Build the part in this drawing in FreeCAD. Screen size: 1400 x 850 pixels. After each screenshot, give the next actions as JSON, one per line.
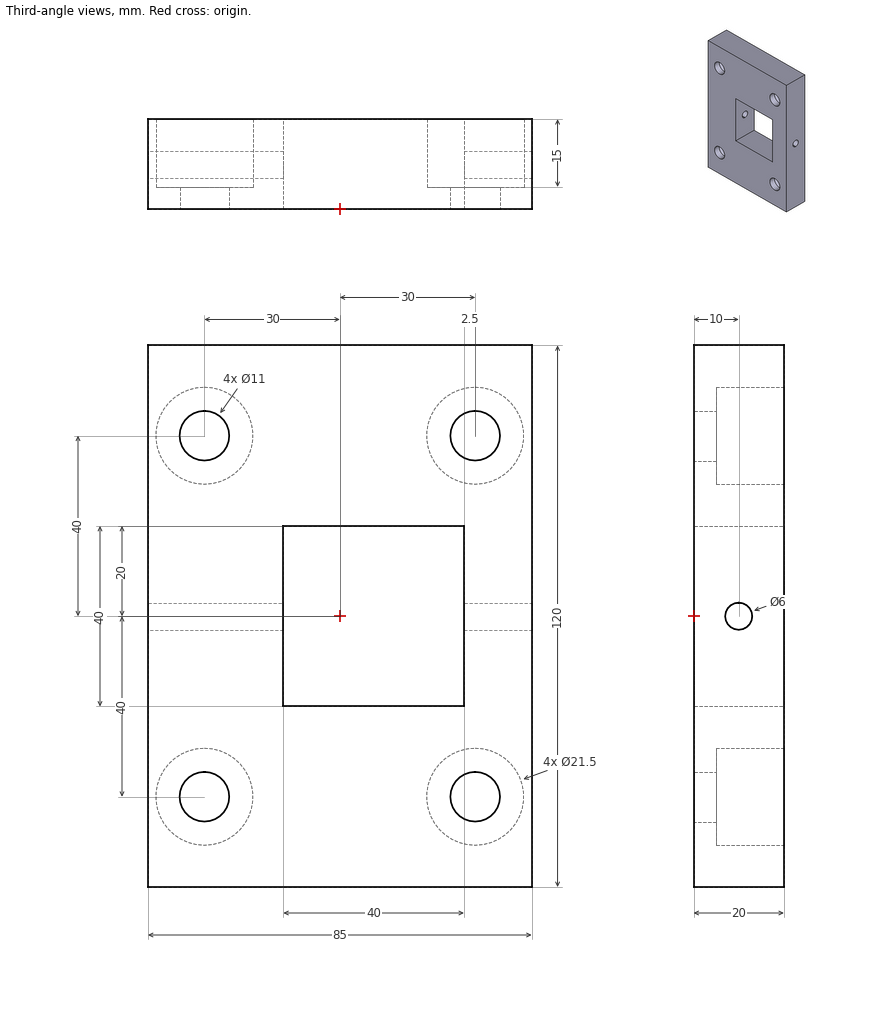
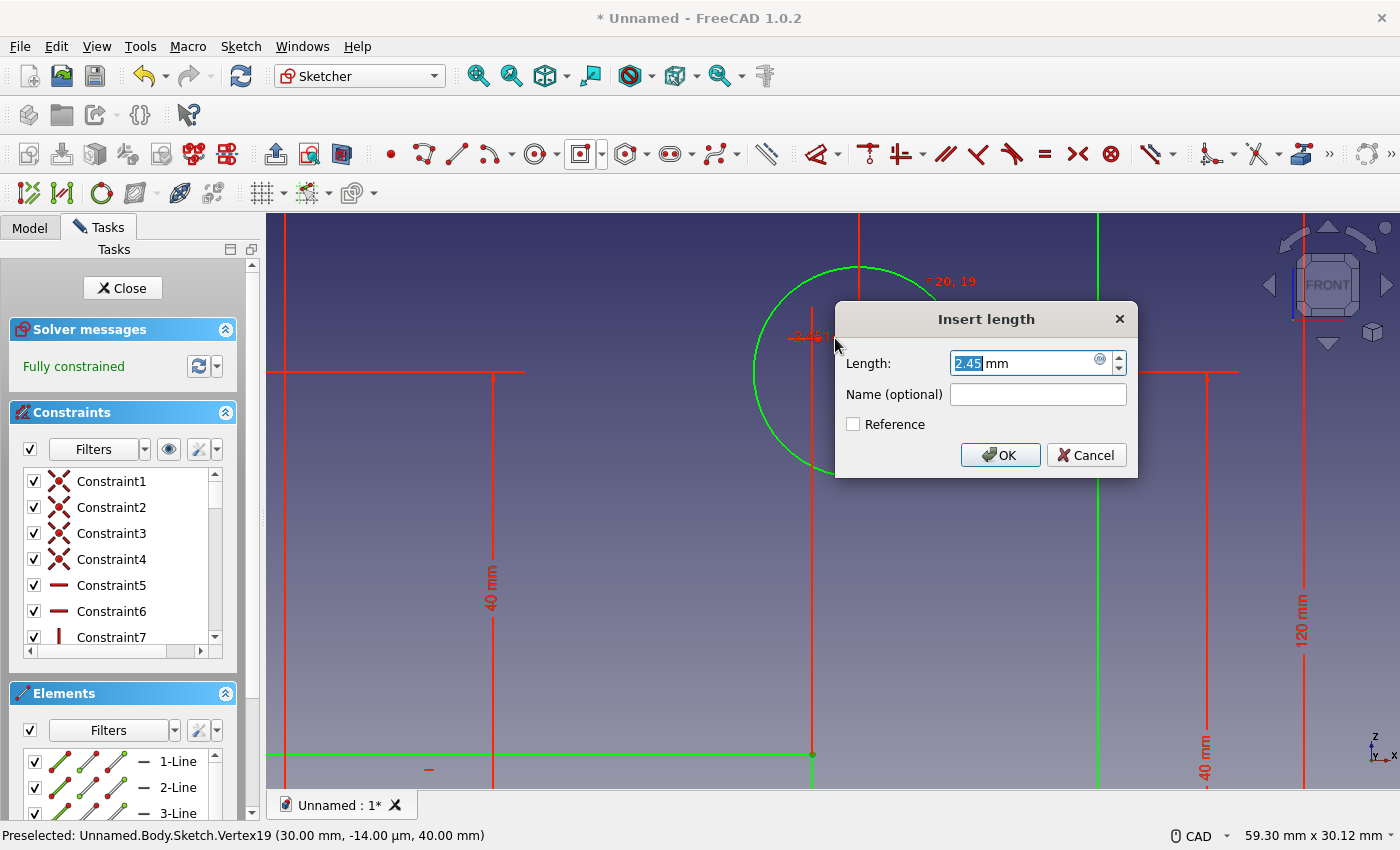
{"action": "type", "text": "2.5"}
{"action": "key", "text": "Return"}
{"action": "key", "text": "Escape"}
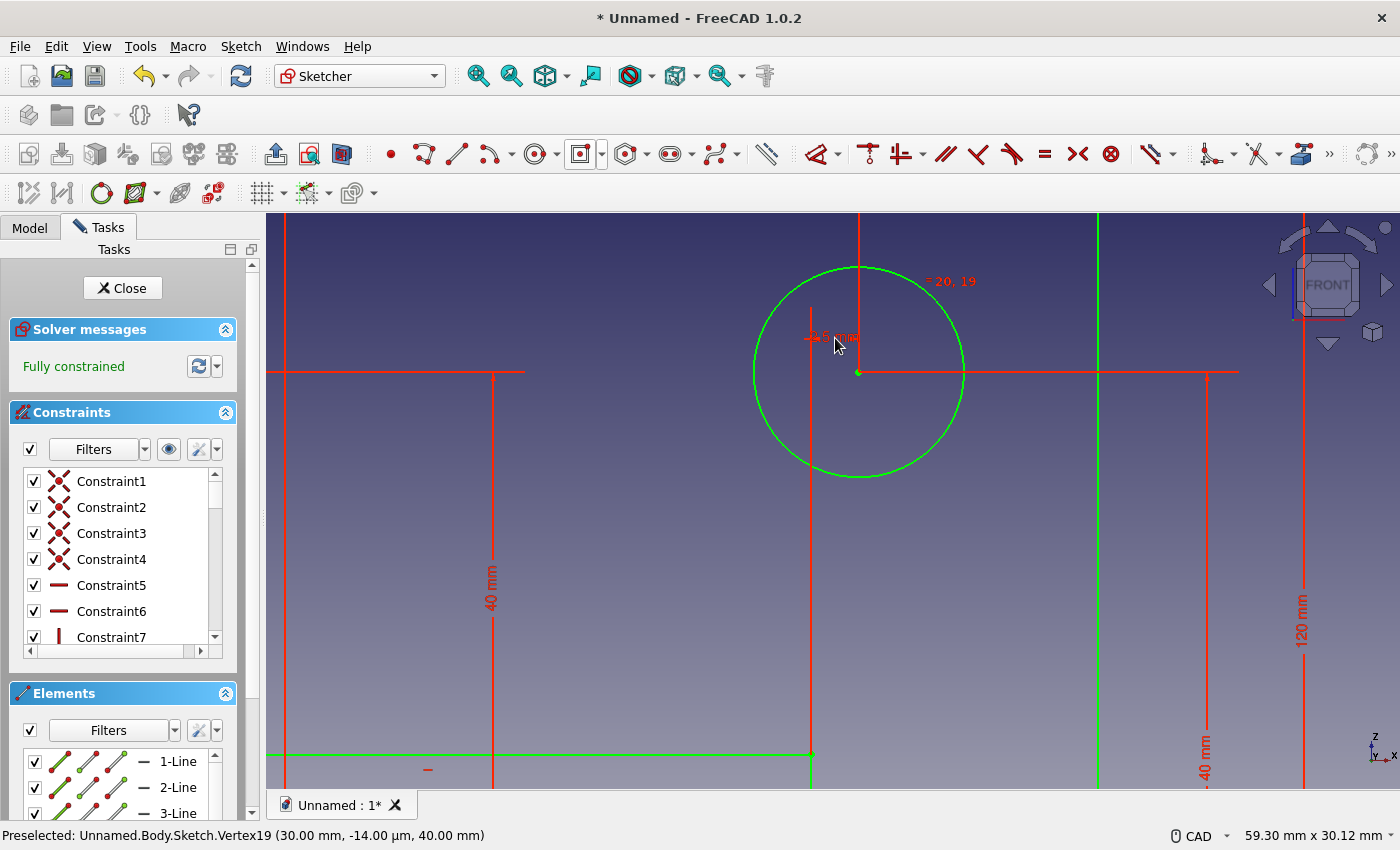
{"action": "left_click", "coordinate": [123, 288]}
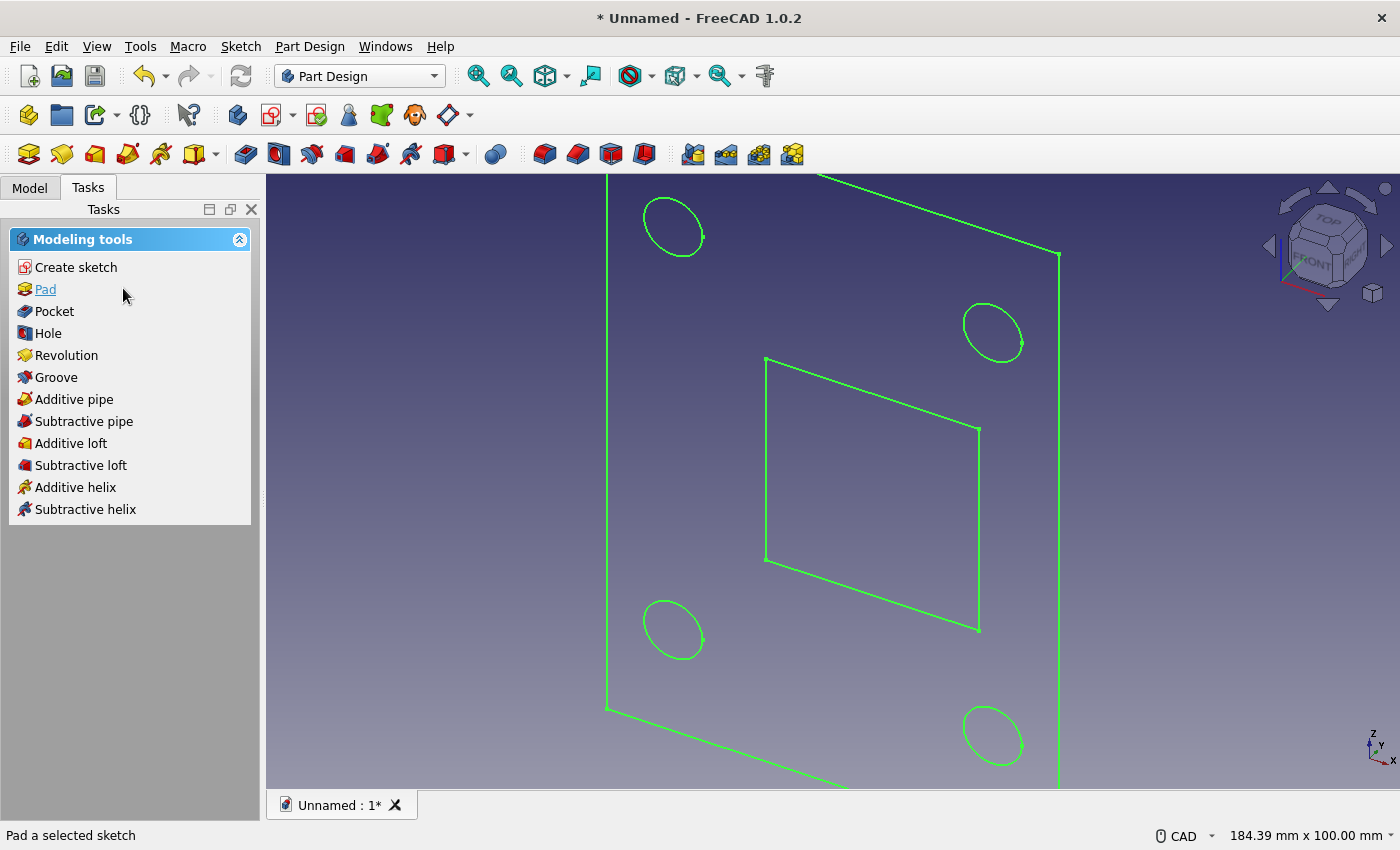
{"action": "left_click", "coordinate": [29, 154]}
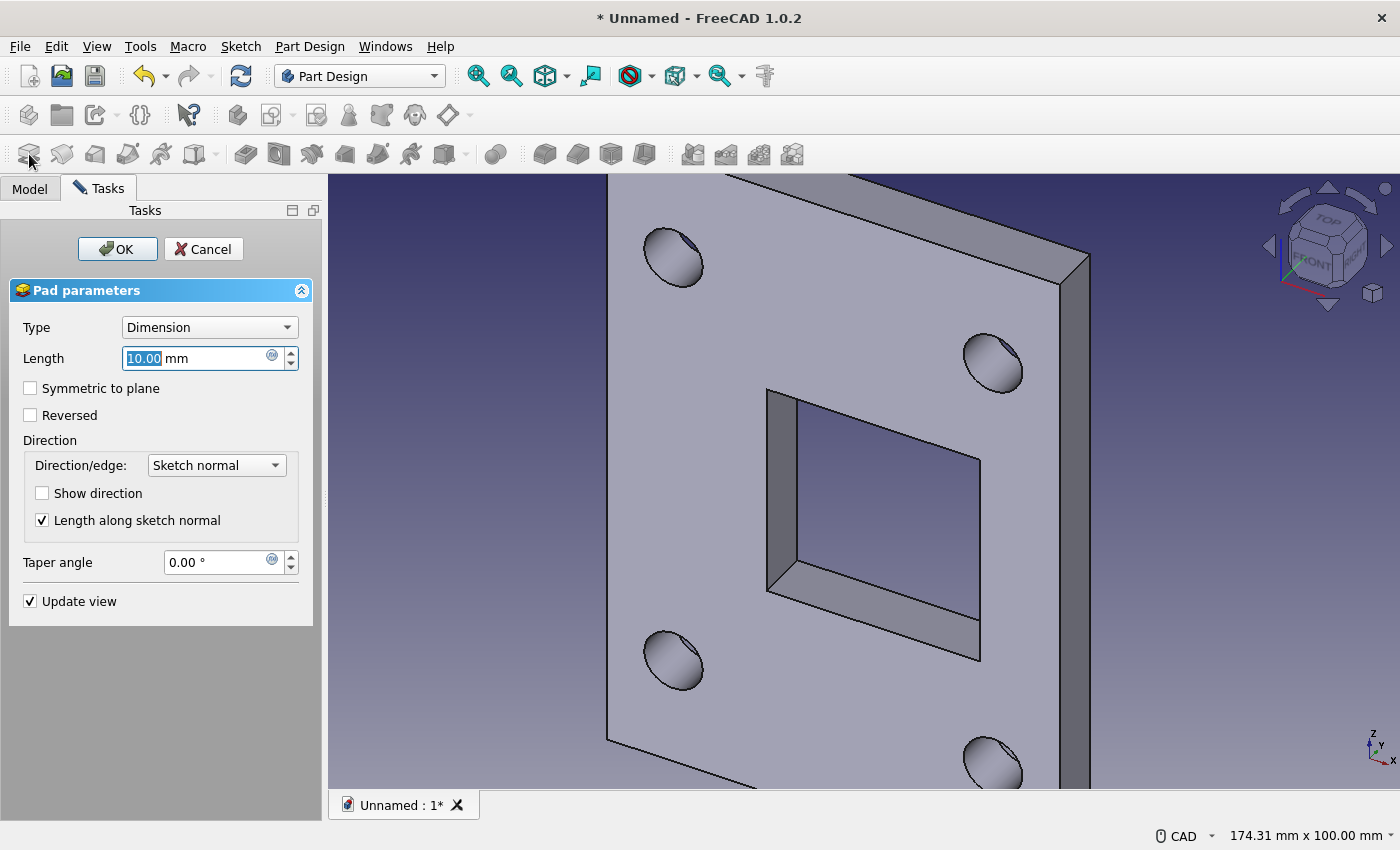
{"action": "type", "text": "20"}
{"action": "key", "text": "Tab"}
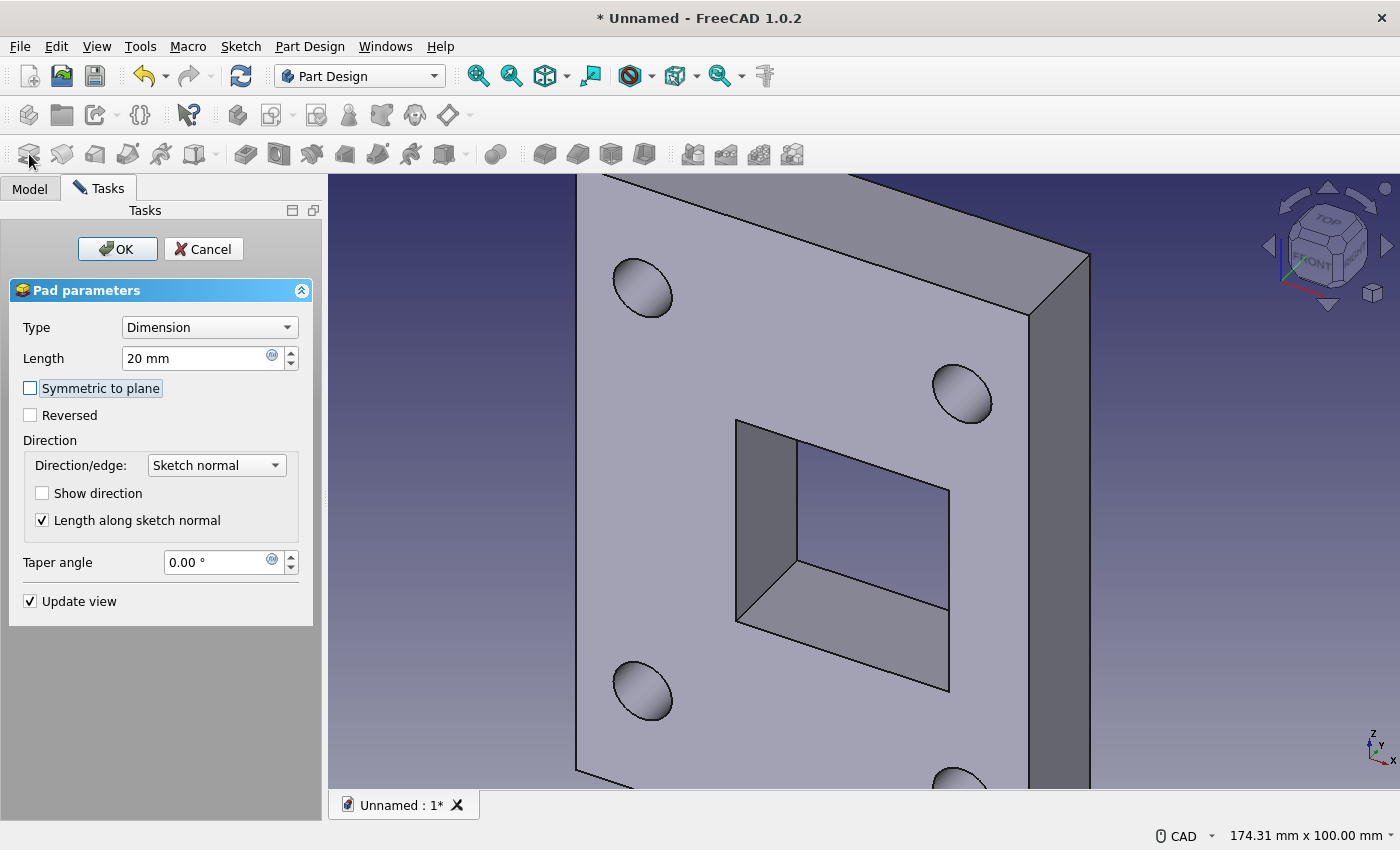
{"action": "left_click", "coordinate": [31, 415]}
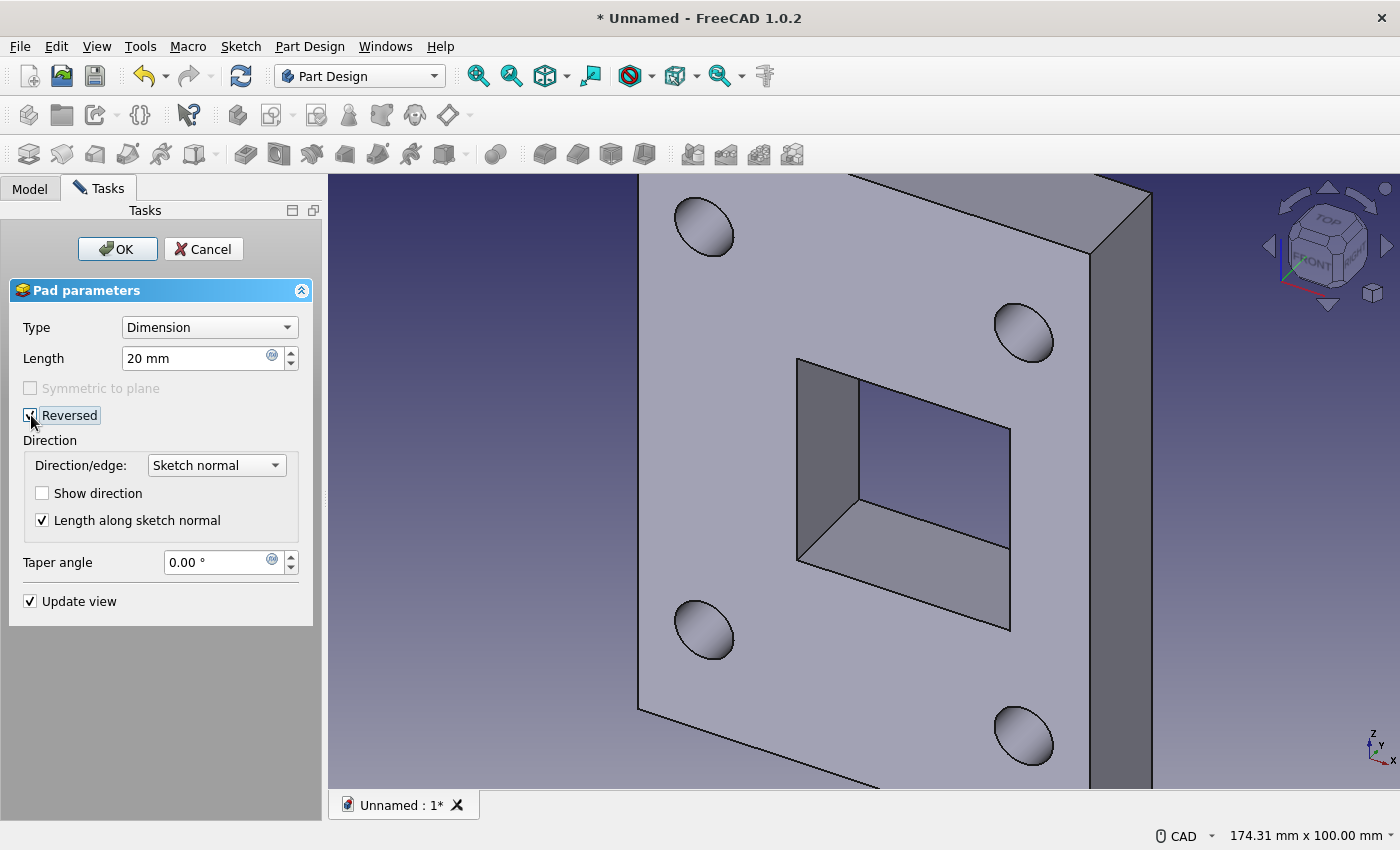
{"action": "left_click", "coordinate": [118, 249]}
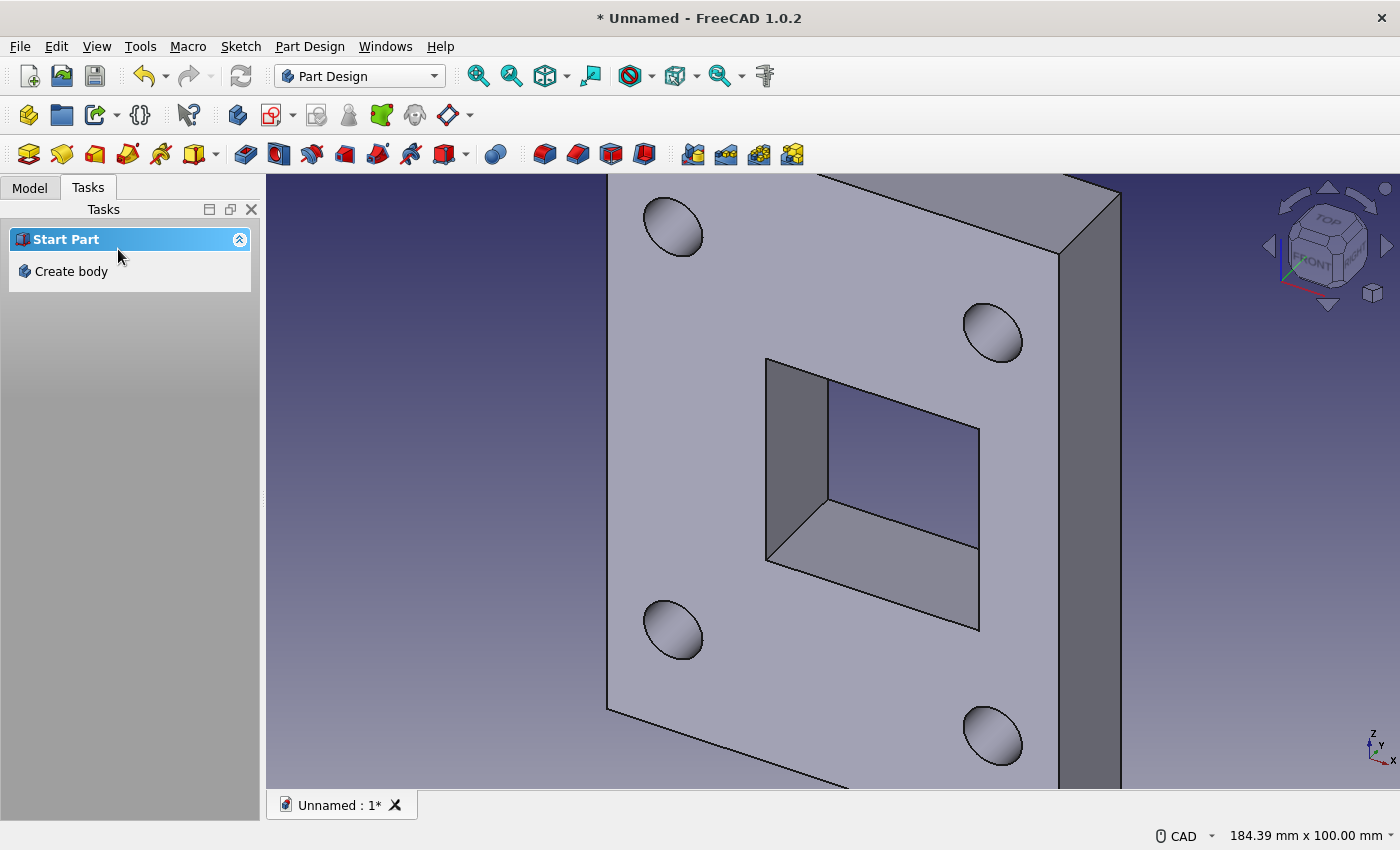
{"action": "left_click", "coordinate": [479, 76]}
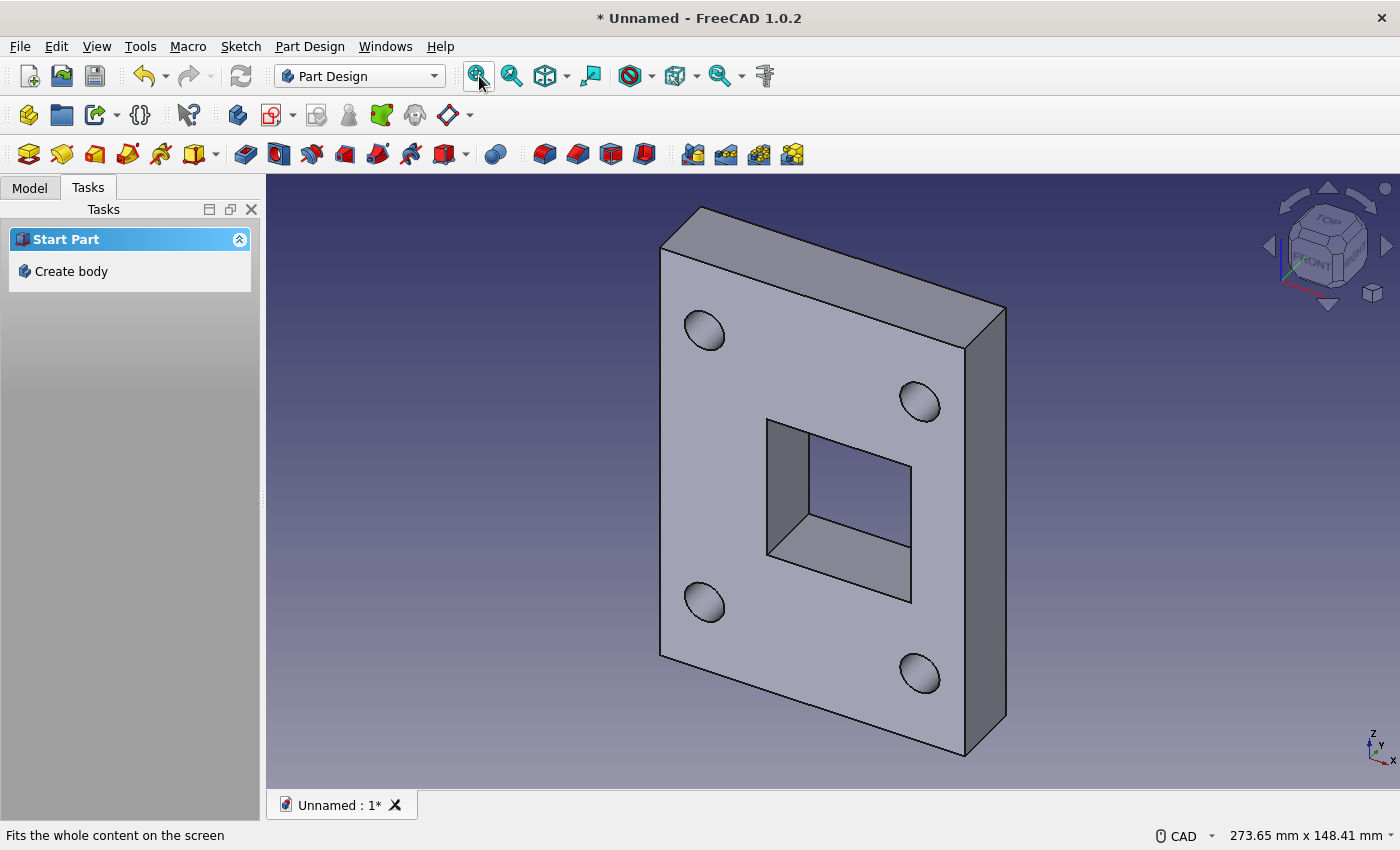
{"action": "key", "text": "4"}